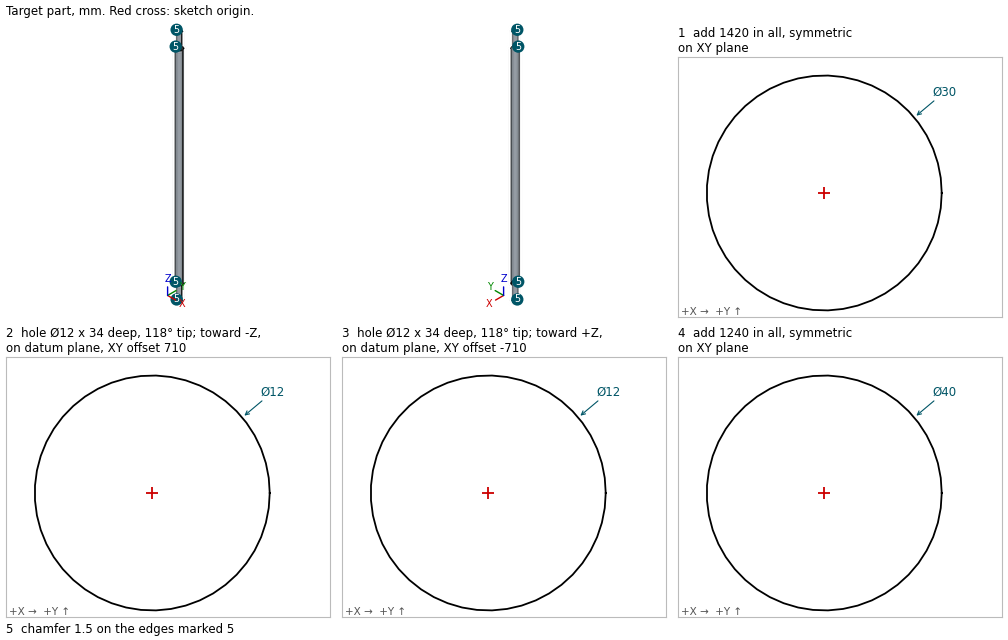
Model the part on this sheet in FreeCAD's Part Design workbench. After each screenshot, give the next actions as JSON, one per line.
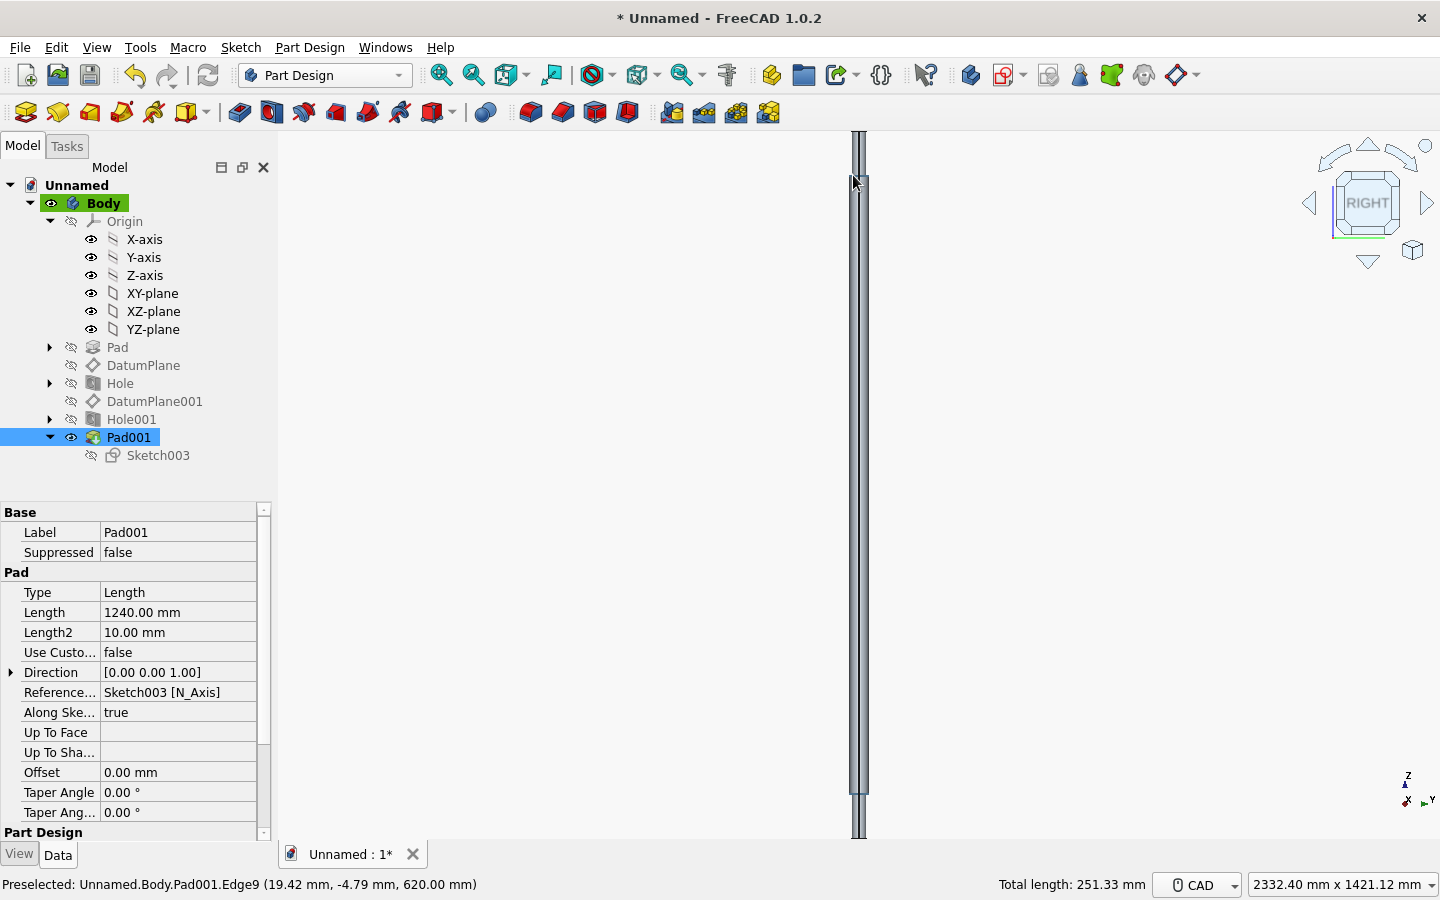
{"action": "key", "text": "0"}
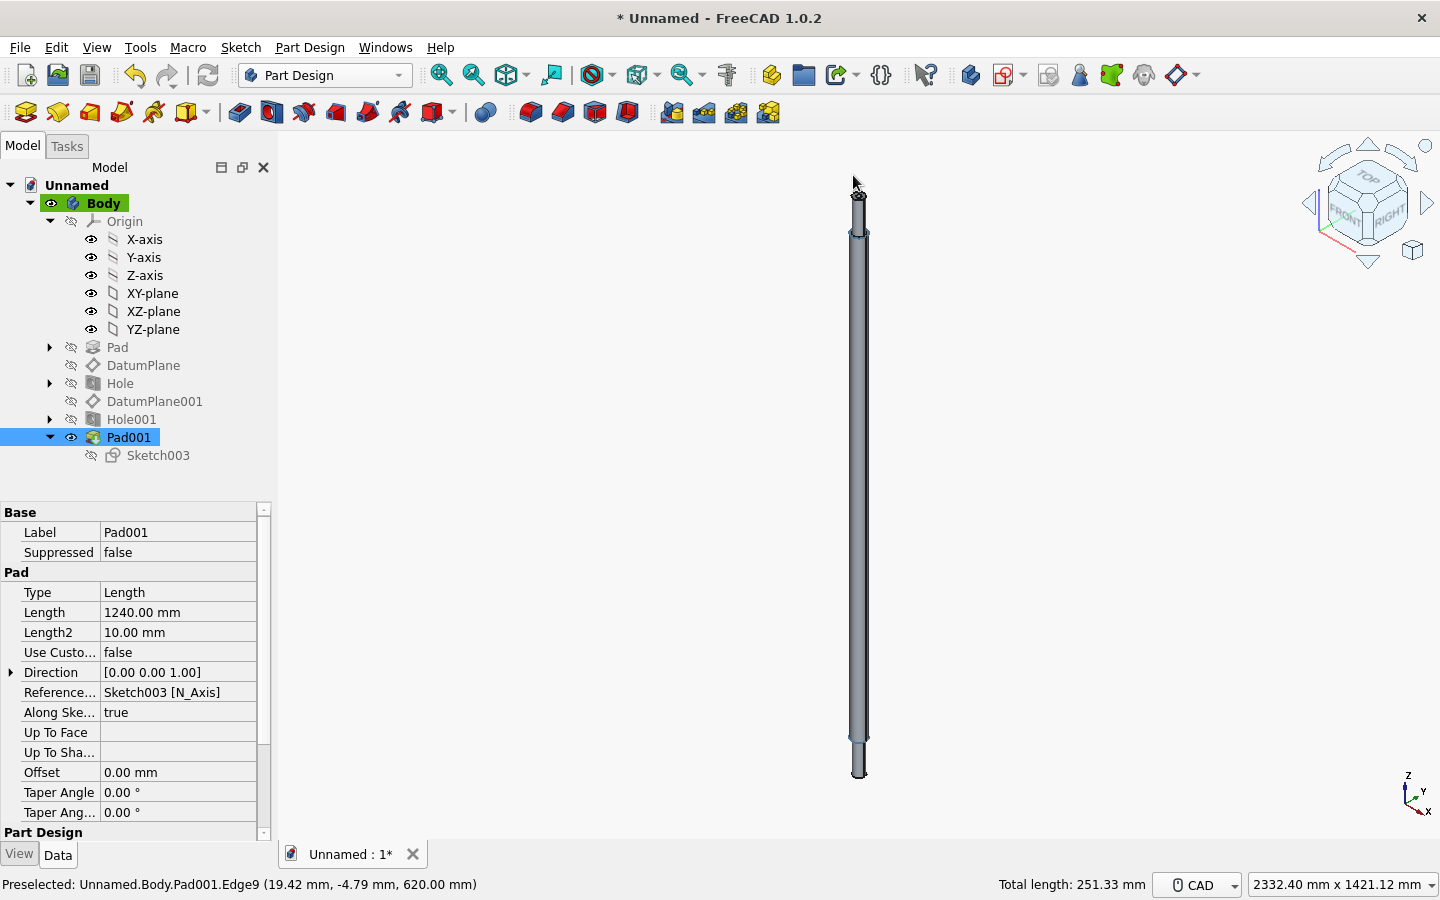
{"action": "left_click", "coordinate": [852, 775], "text": "ctrl"}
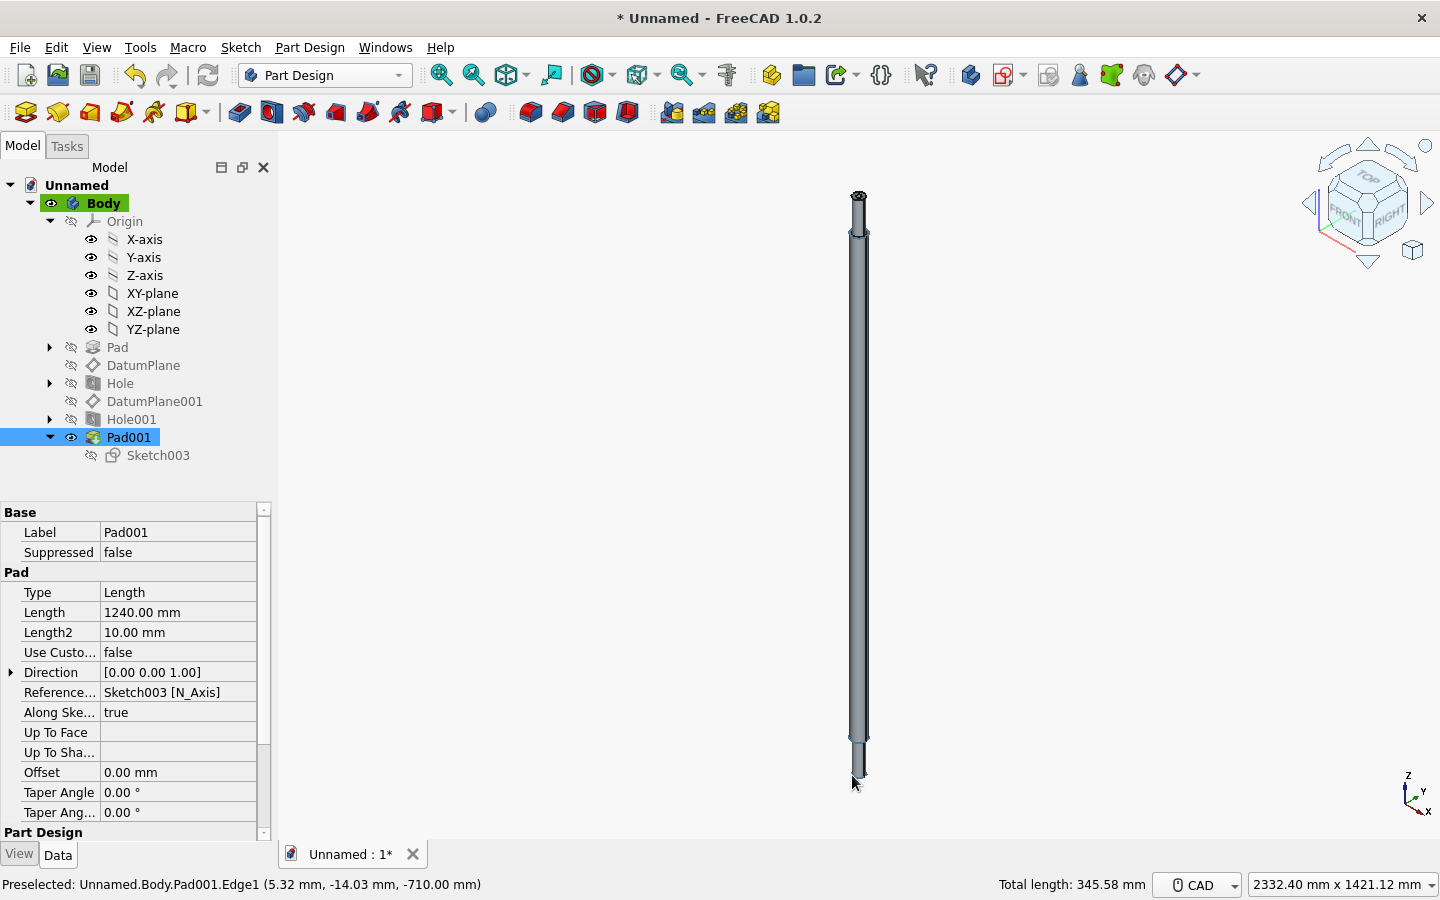
{"action": "left_click", "coordinate": [852, 195], "text": "ctrl"}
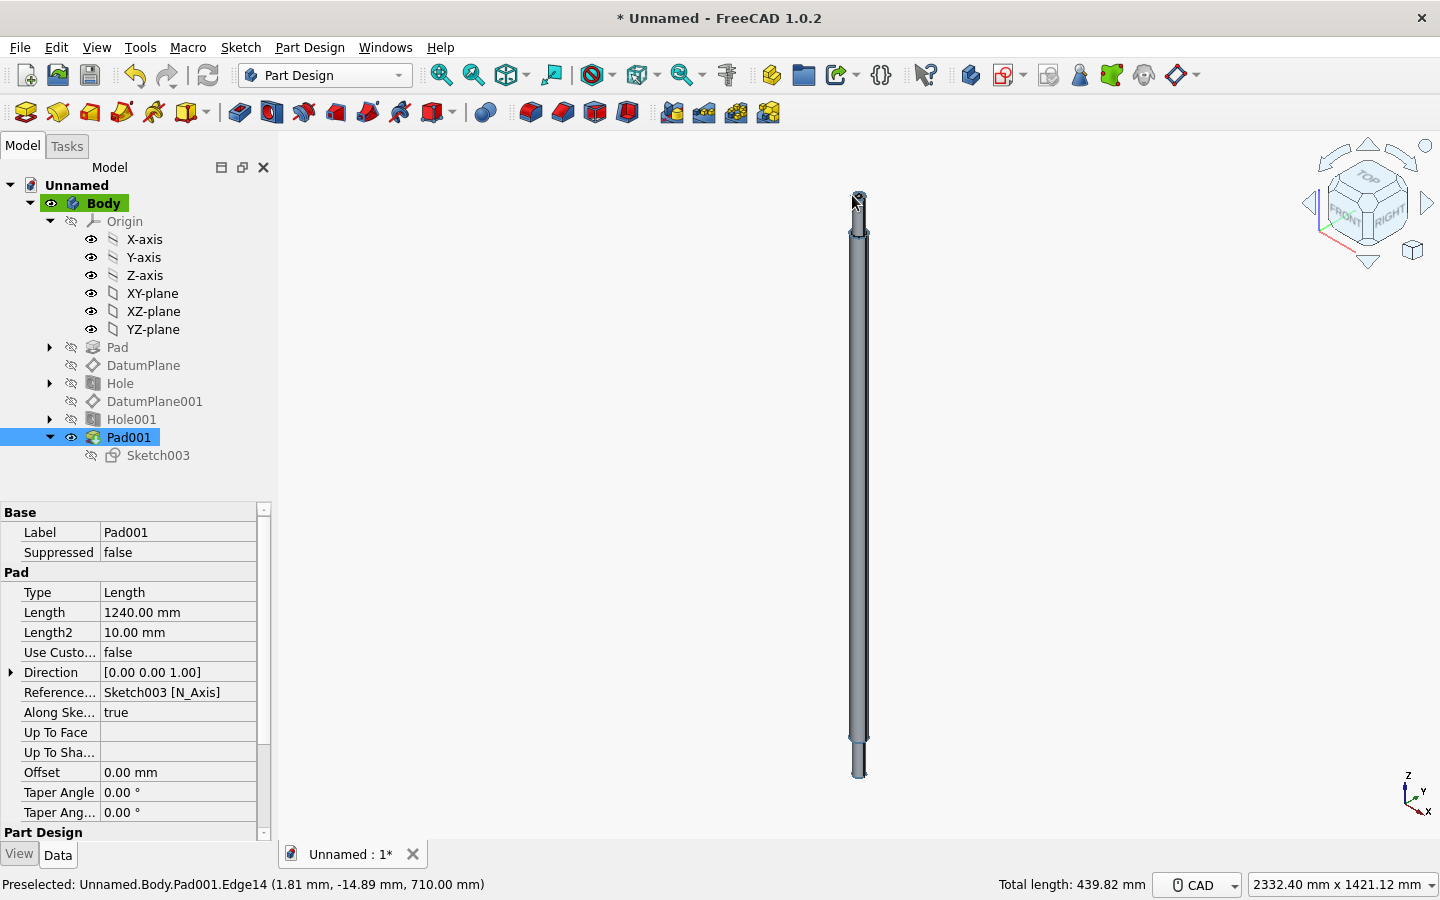
{"action": "left_click", "coordinate": [564, 112]}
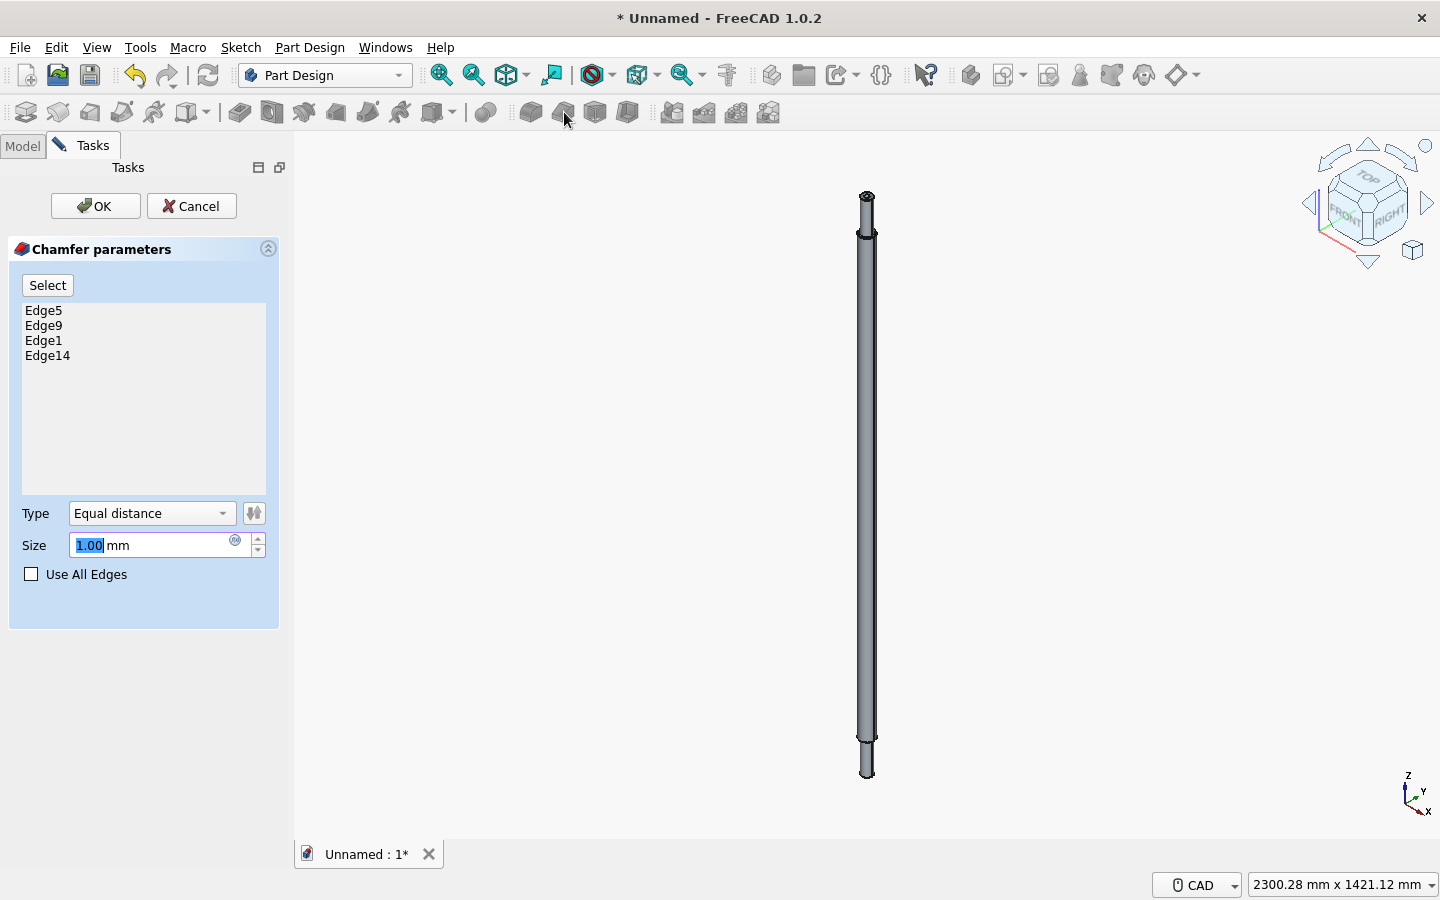
{"action": "type", "text": "1.5"}
{"action": "key", "text": "Tab"}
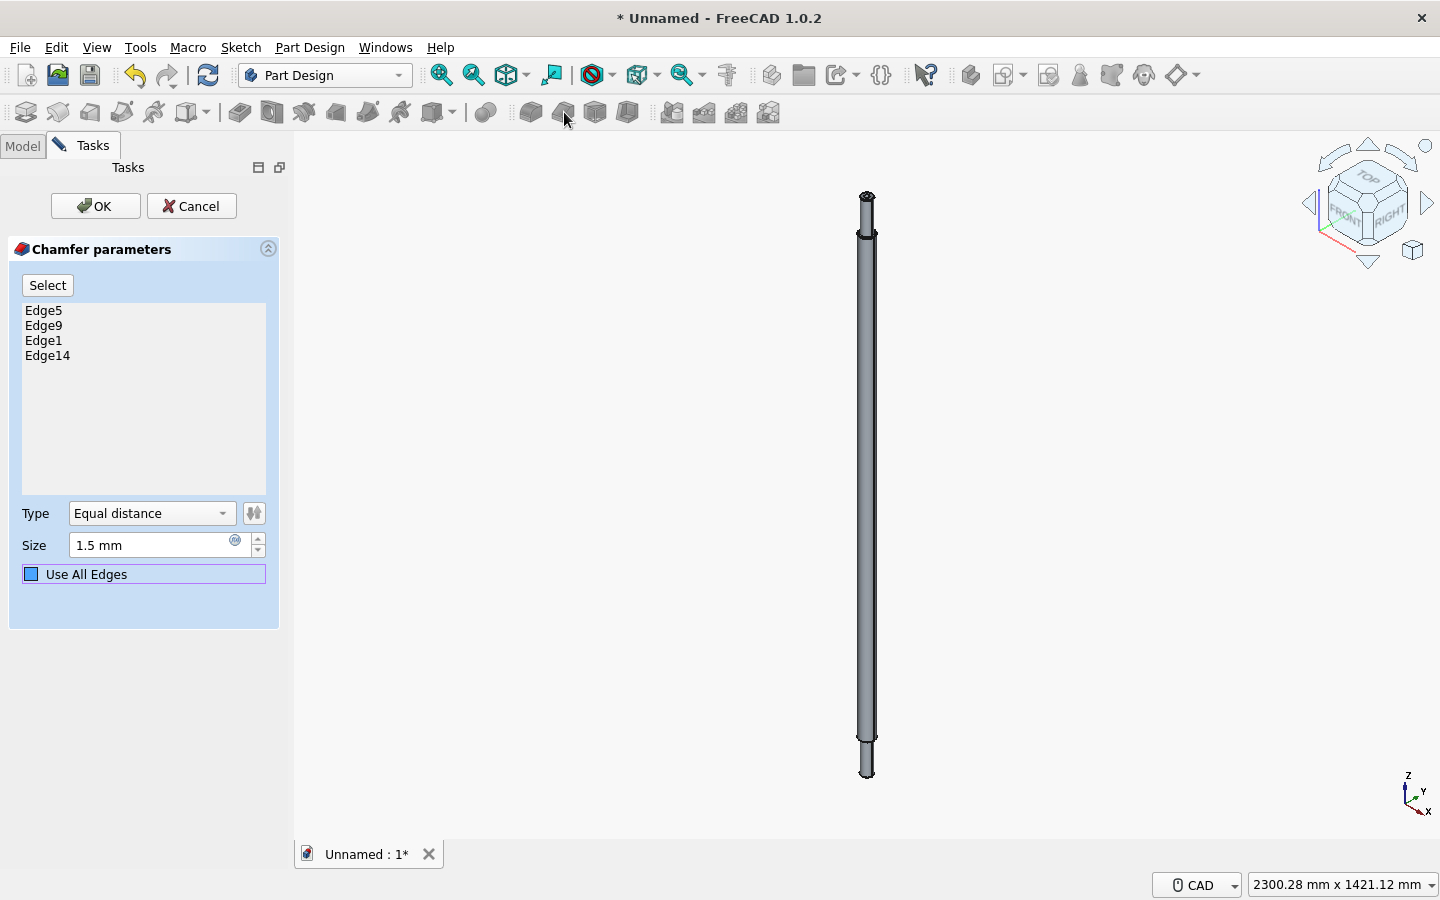
{"action": "left_click", "coordinate": [96, 206]}